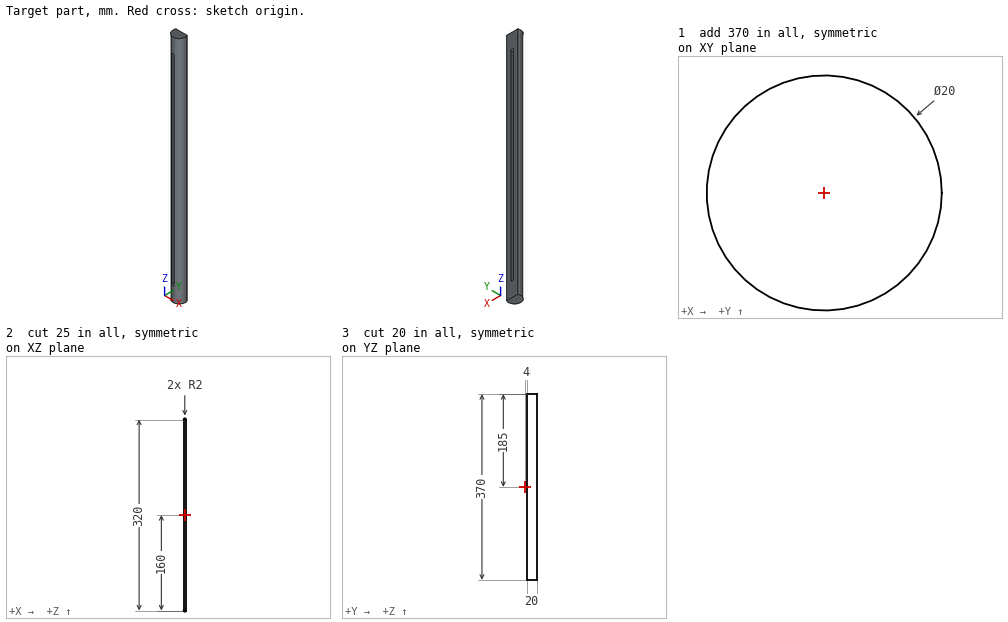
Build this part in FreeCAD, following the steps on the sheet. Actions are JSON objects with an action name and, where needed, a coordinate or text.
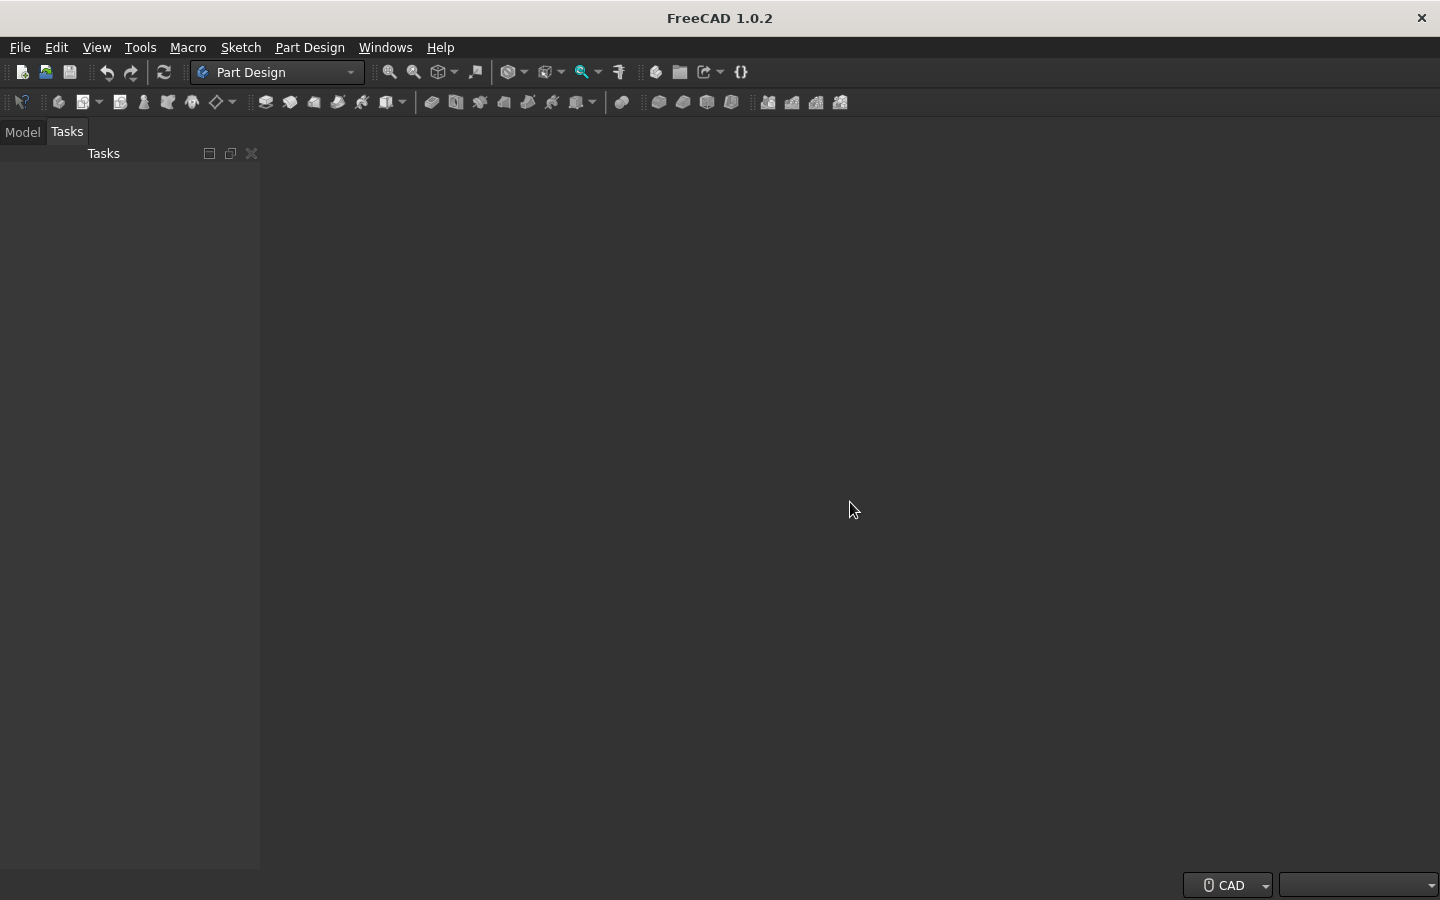
{"action": "left_click", "coordinate": [22, 72]}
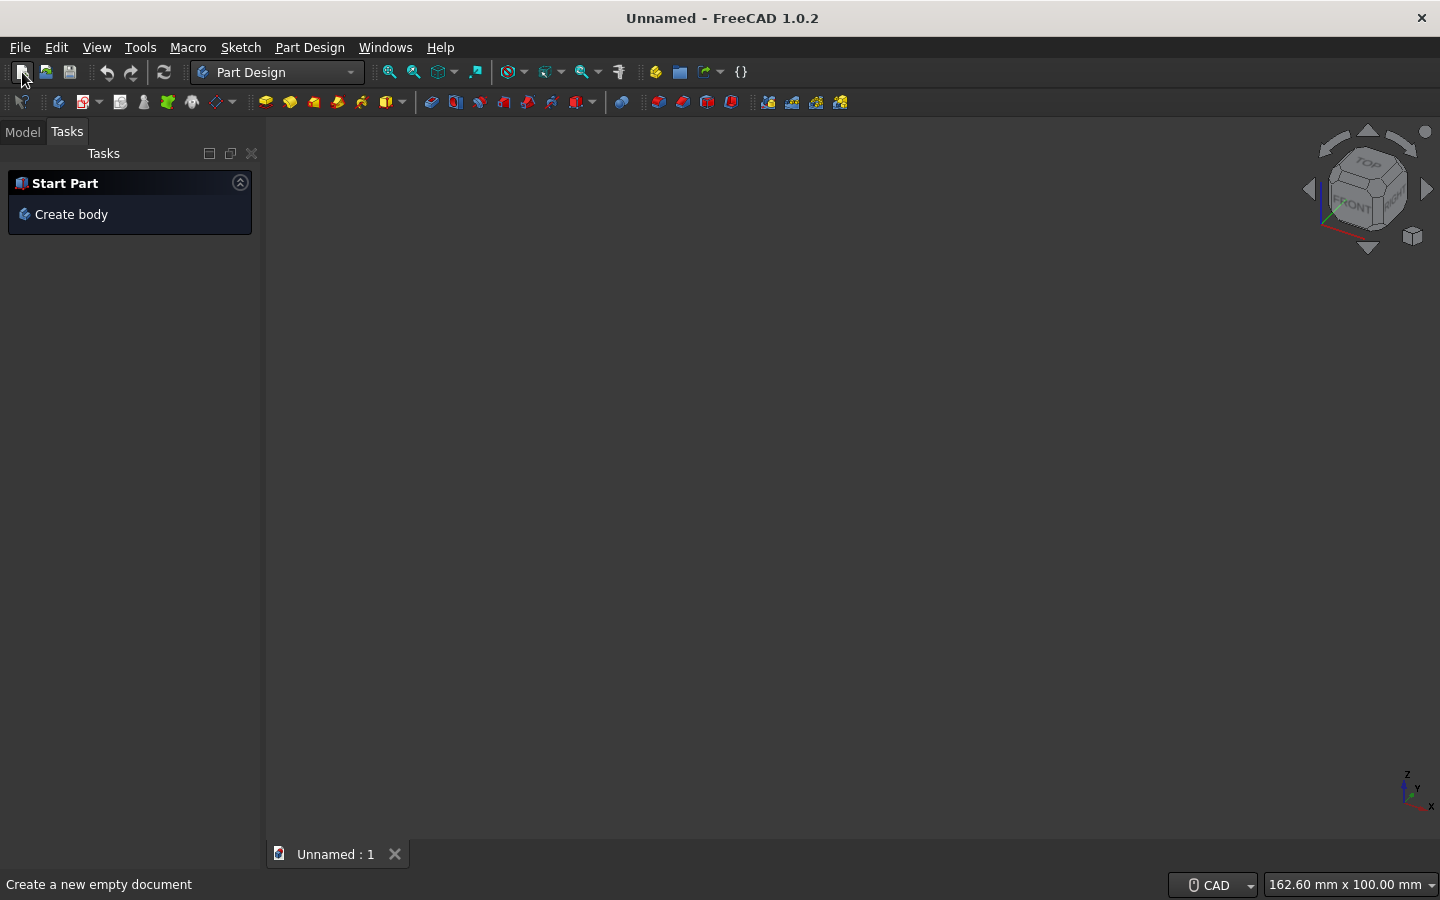
{"action": "left_click", "coordinate": [84, 102]}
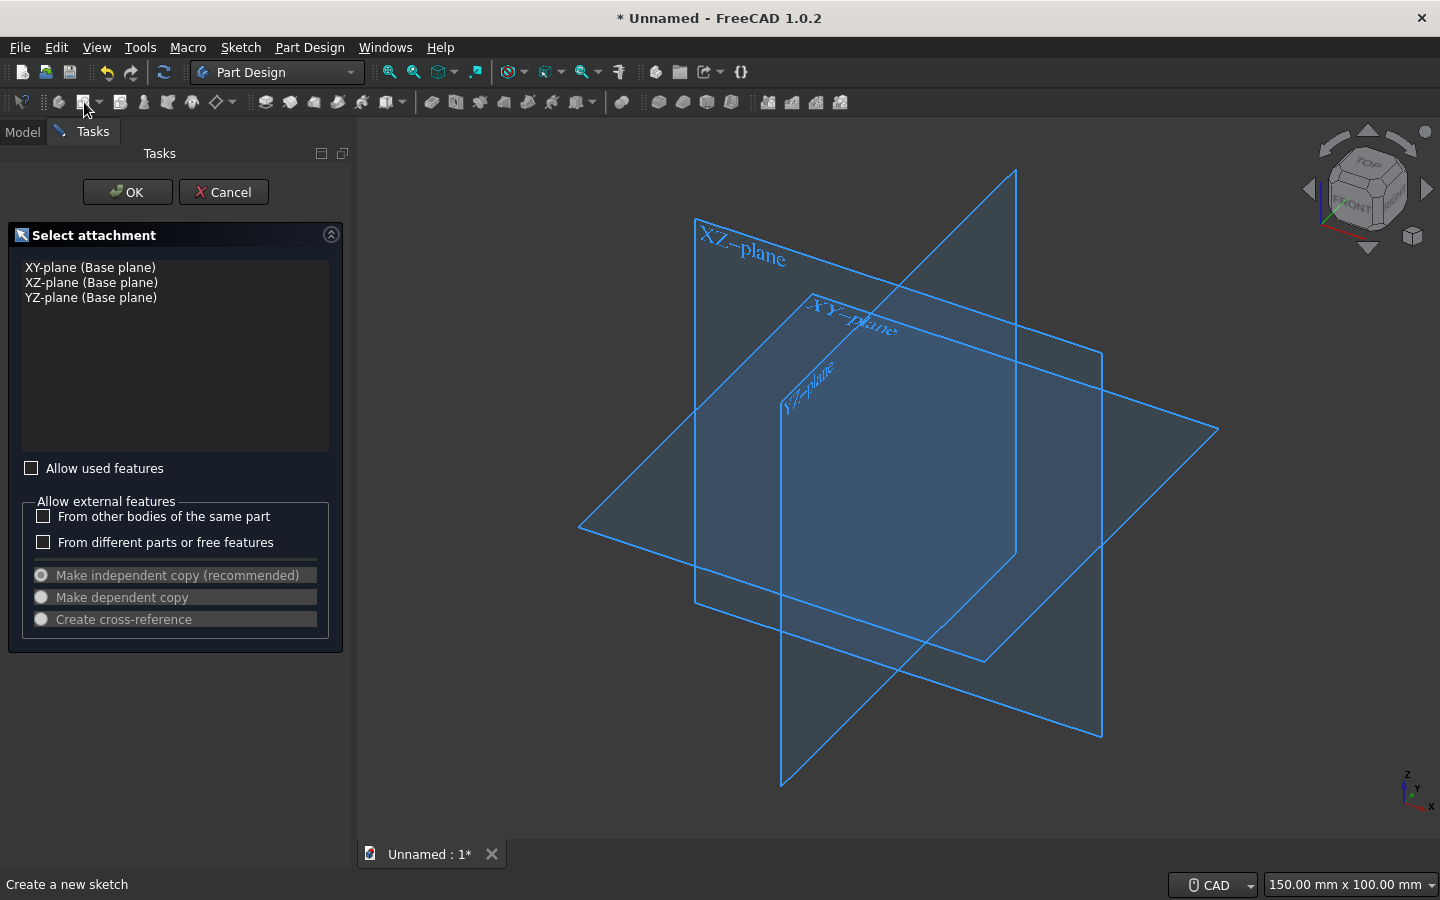
{"action": "left_click", "coordinate": [82, 268]}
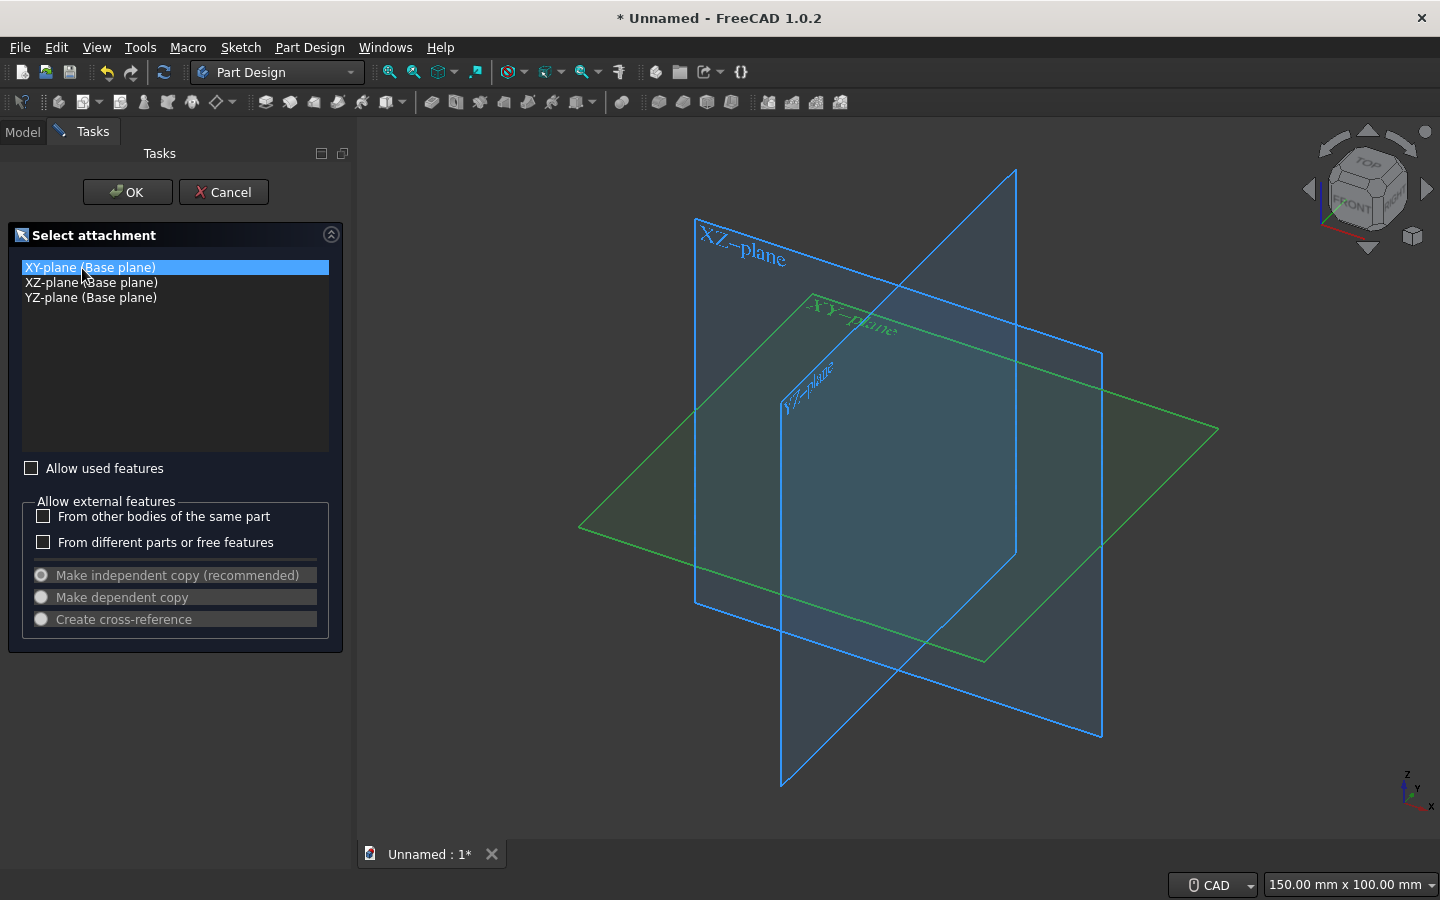
{"action": "left_click", "coordinate": [128, 192]}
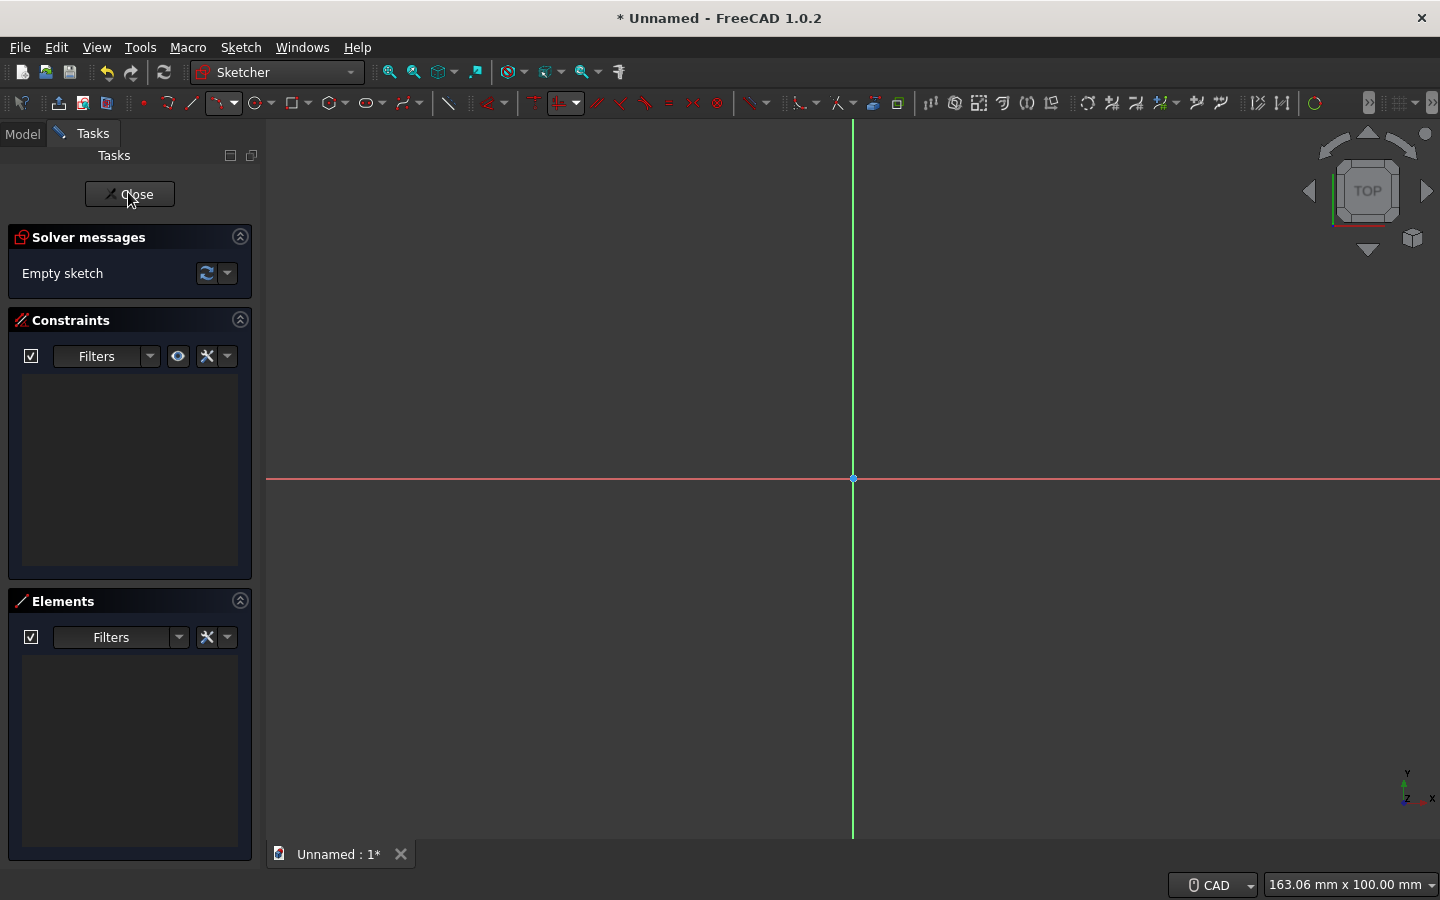
{"action": "scroll", "coordinate": [883, 479], "scroll_direction": "up", "scroll_amount": 6}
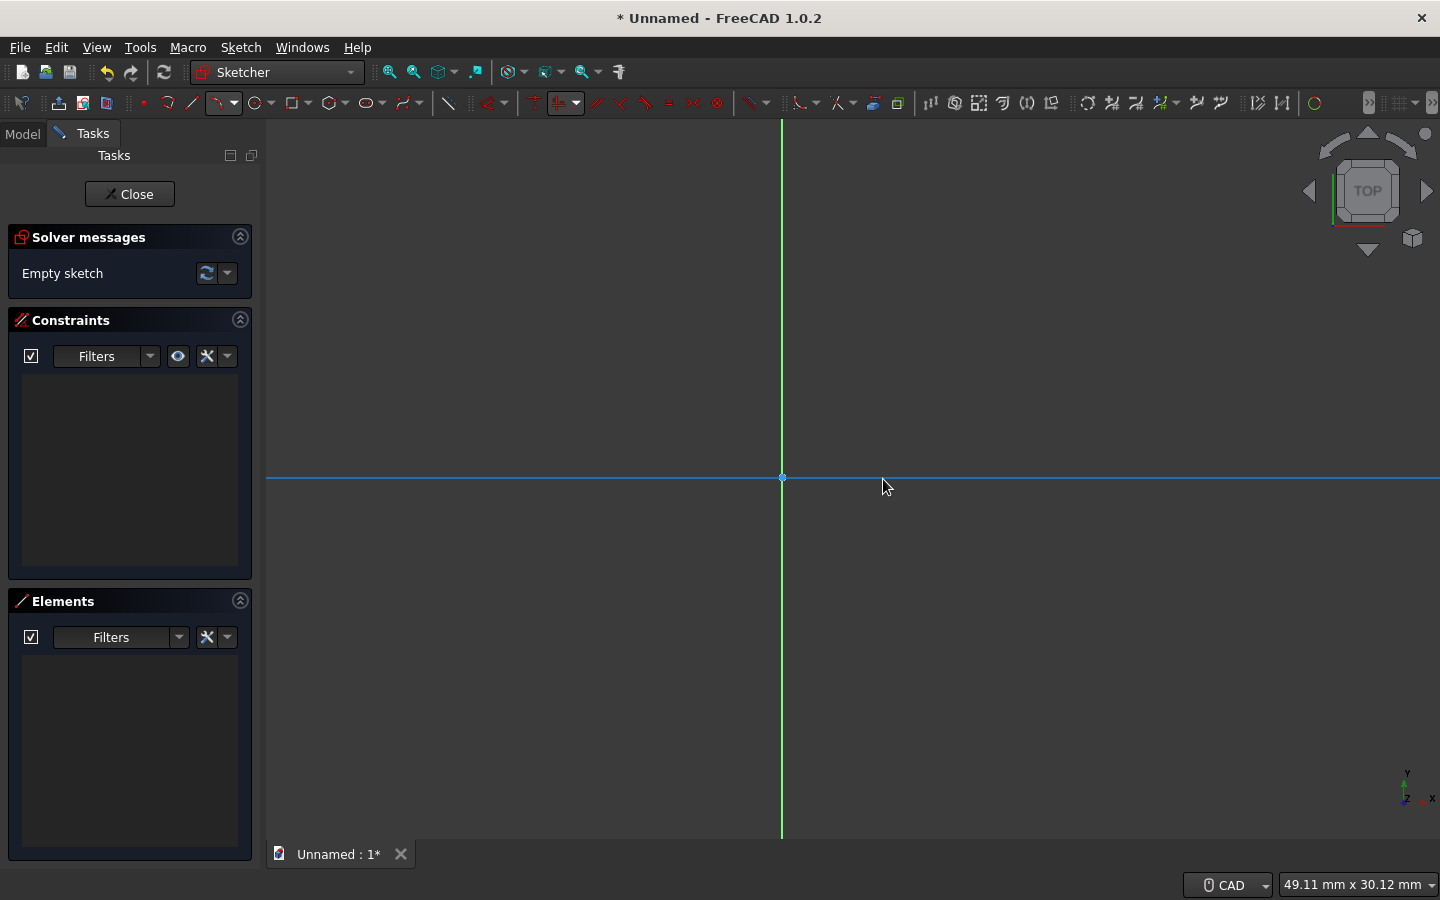
{"action": "left_click", "coordinate": [256, 104]}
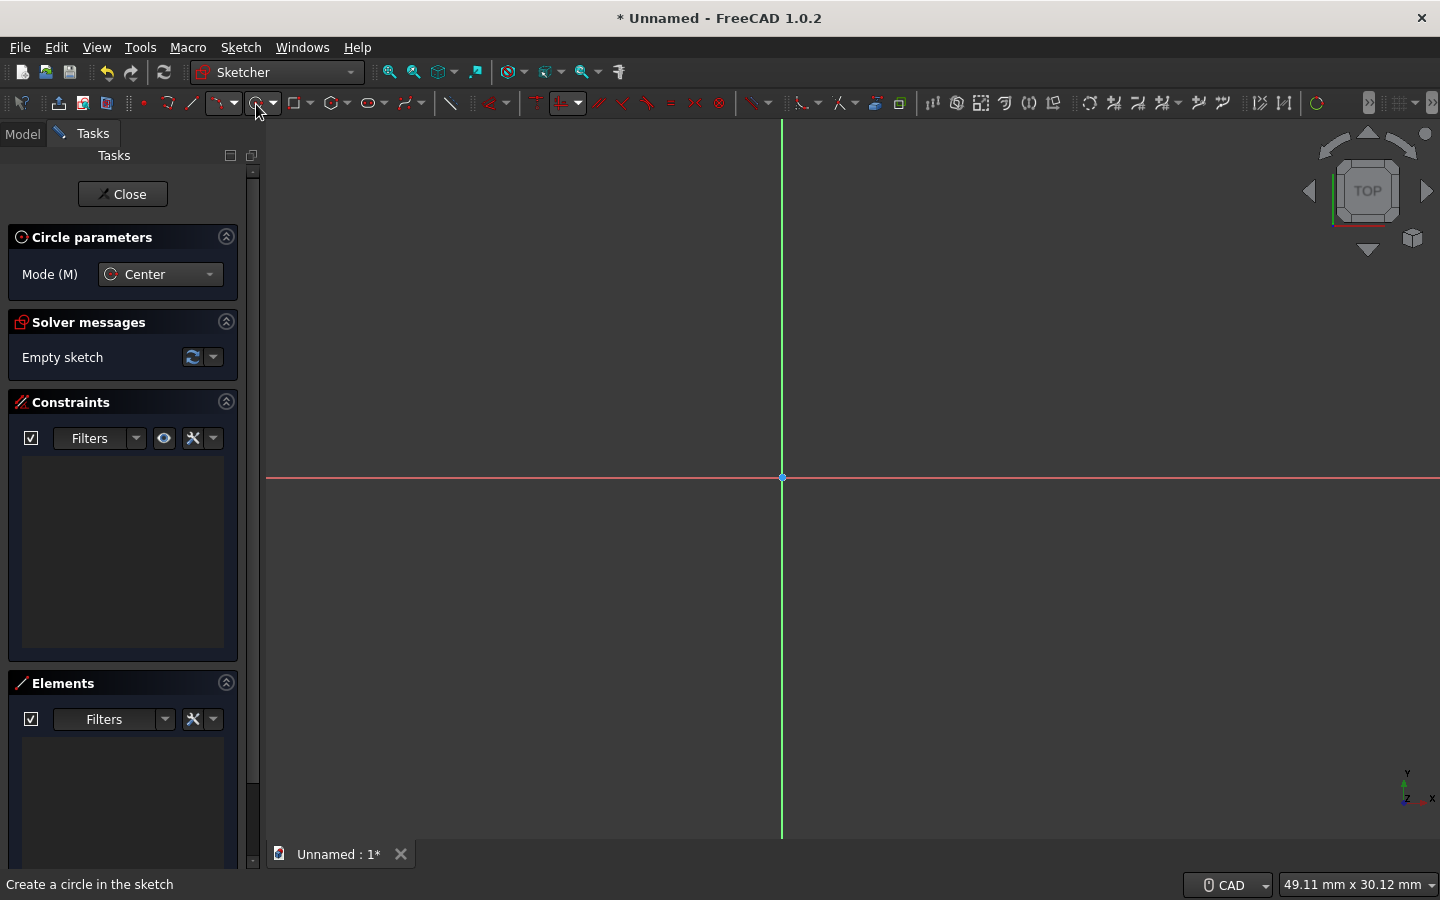
{"action": "left_click", "coordinate": [782, 478]}
{"action": "mouse_move", "coordinate": [951, 309]}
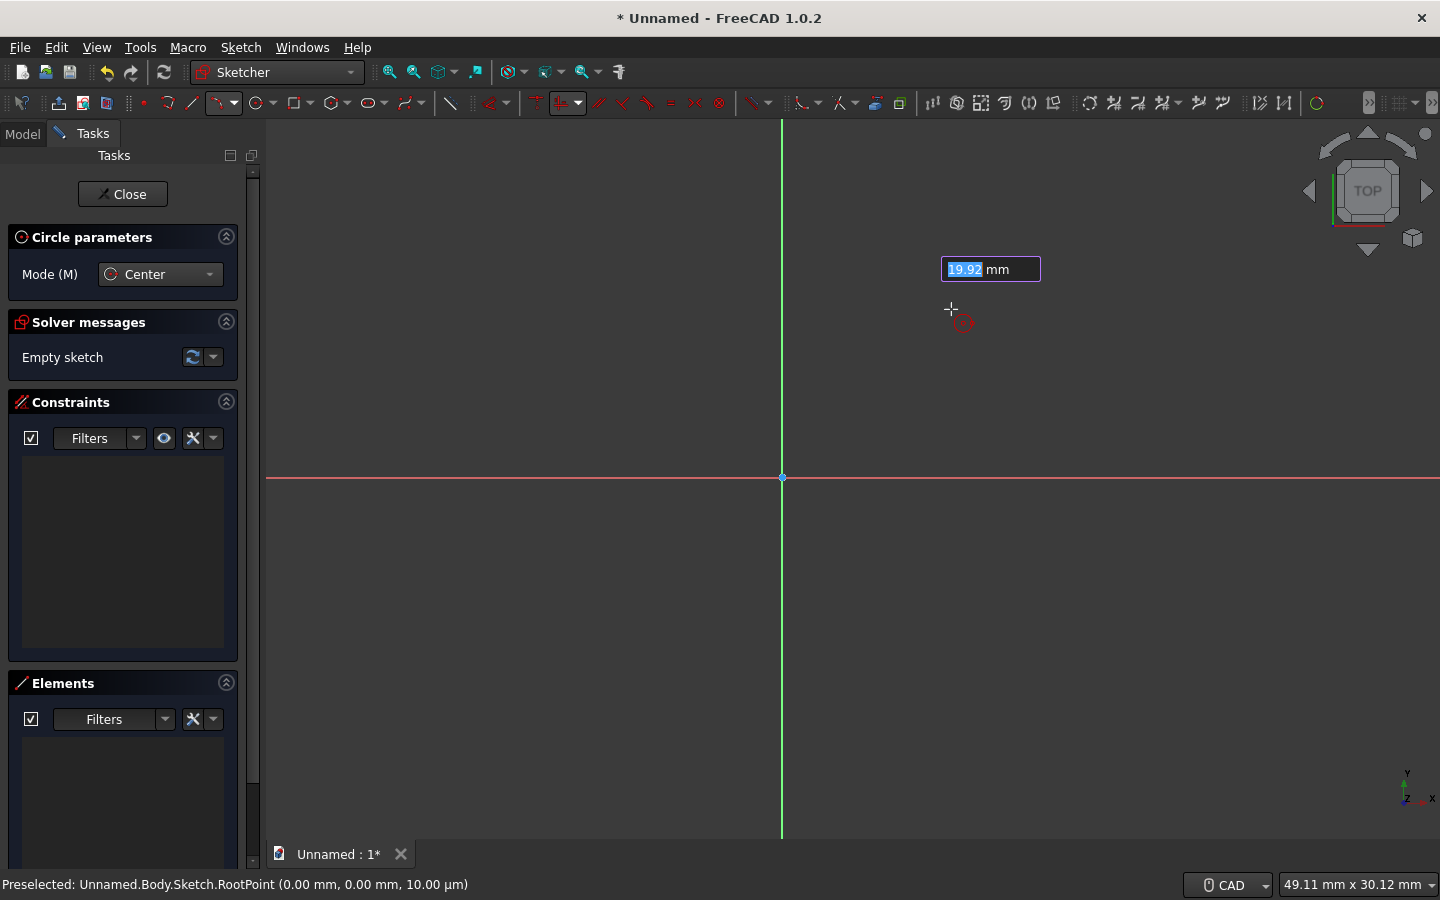
{"action": "type", "text": "20"}
{"action": "key", "text": "Return"}
{"action": "key", "text": "Escape"}